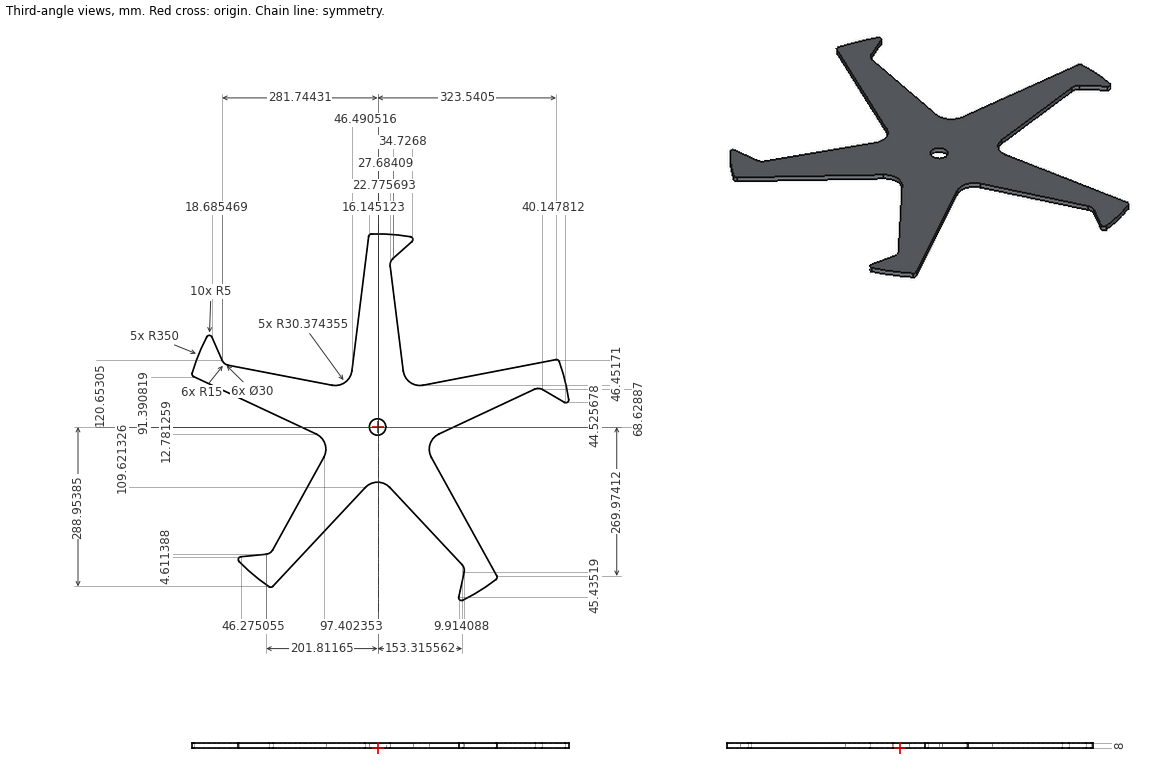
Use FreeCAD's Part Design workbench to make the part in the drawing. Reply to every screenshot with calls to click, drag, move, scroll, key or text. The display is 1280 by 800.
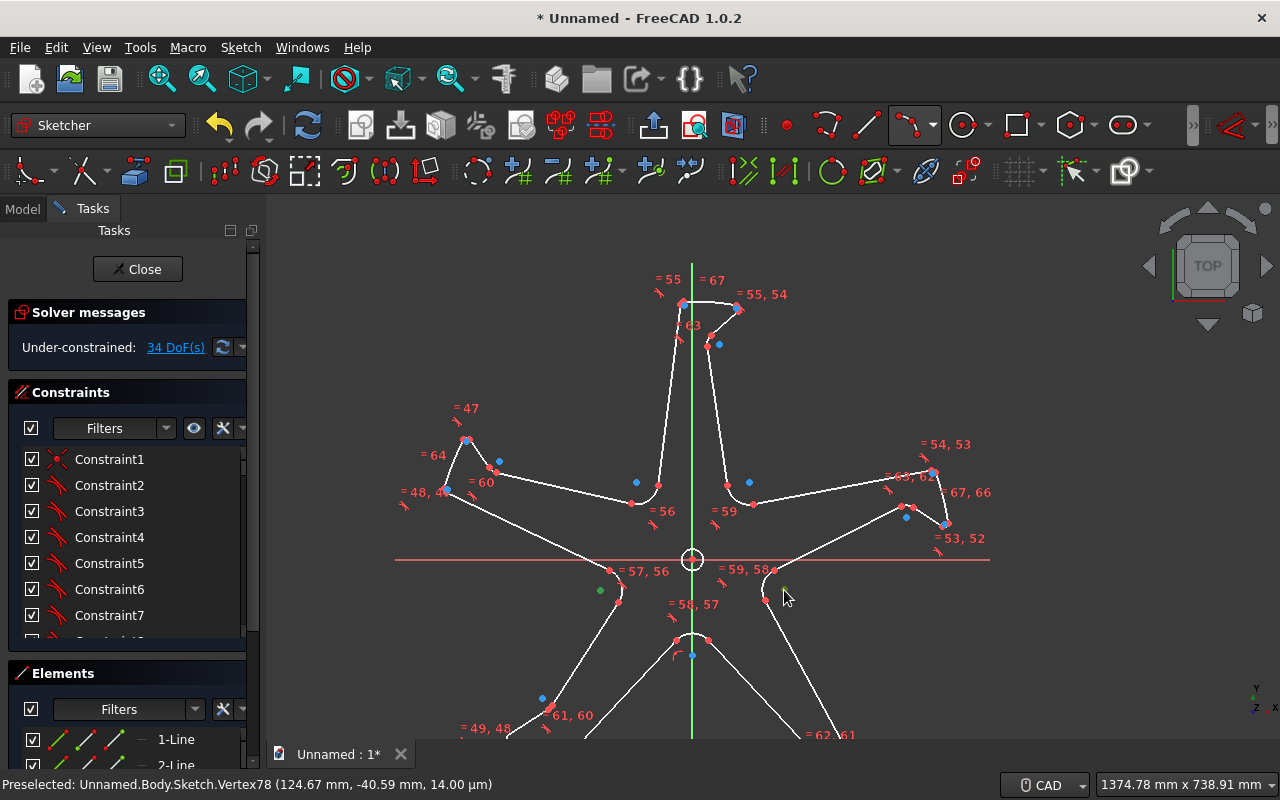
click(692, 676)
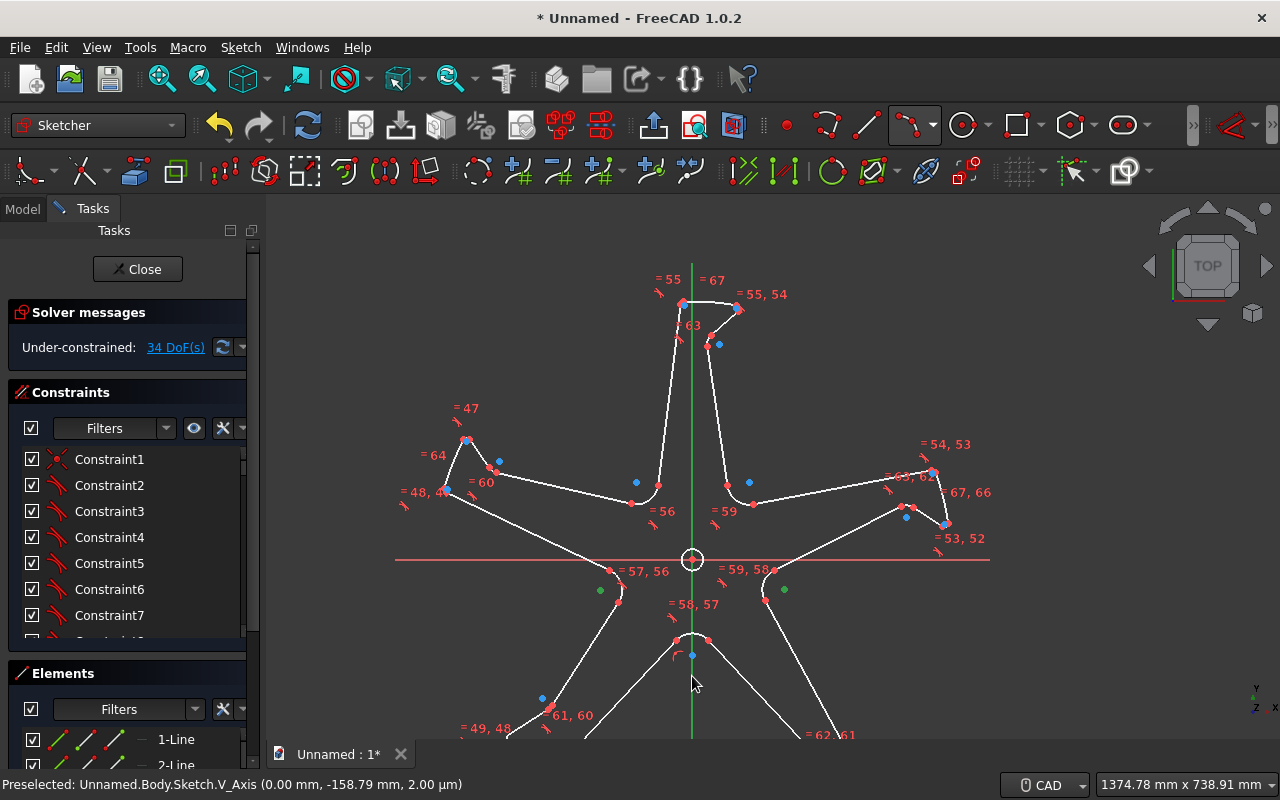
key(s)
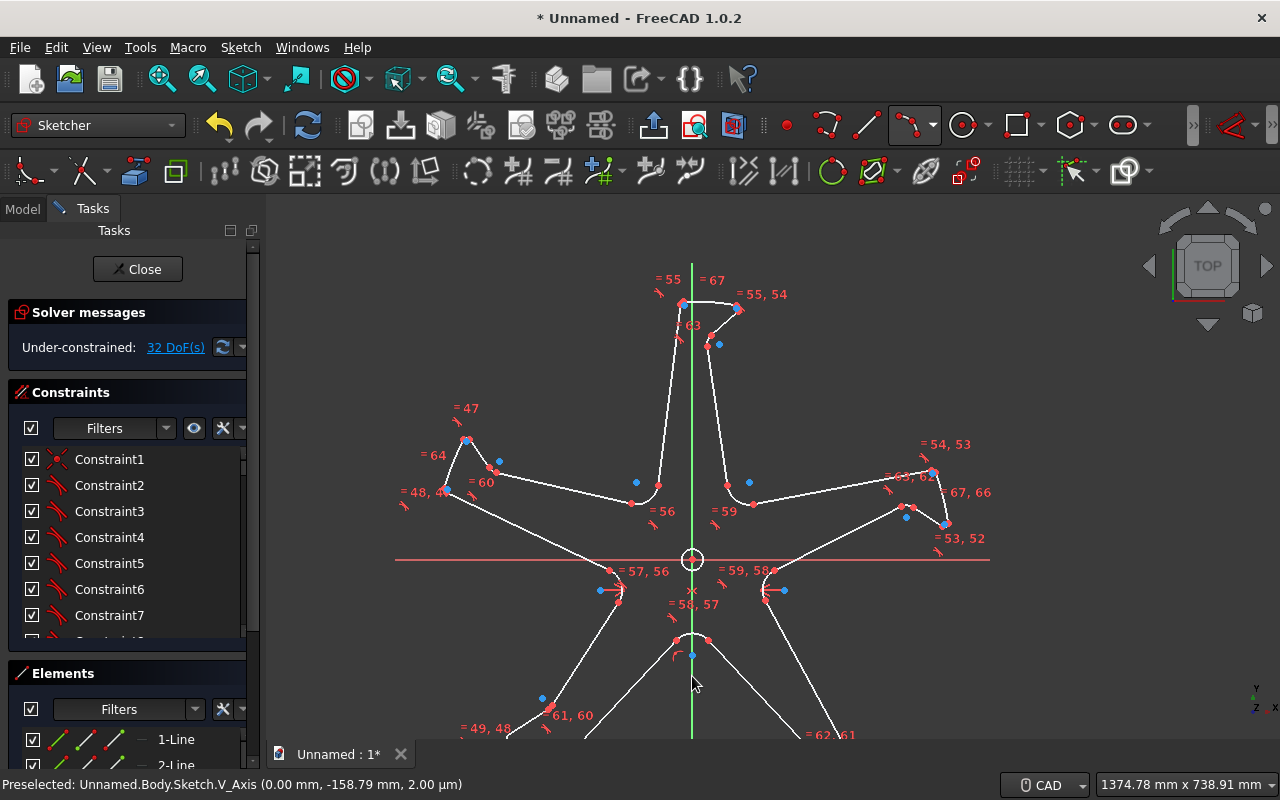
click(636, 482)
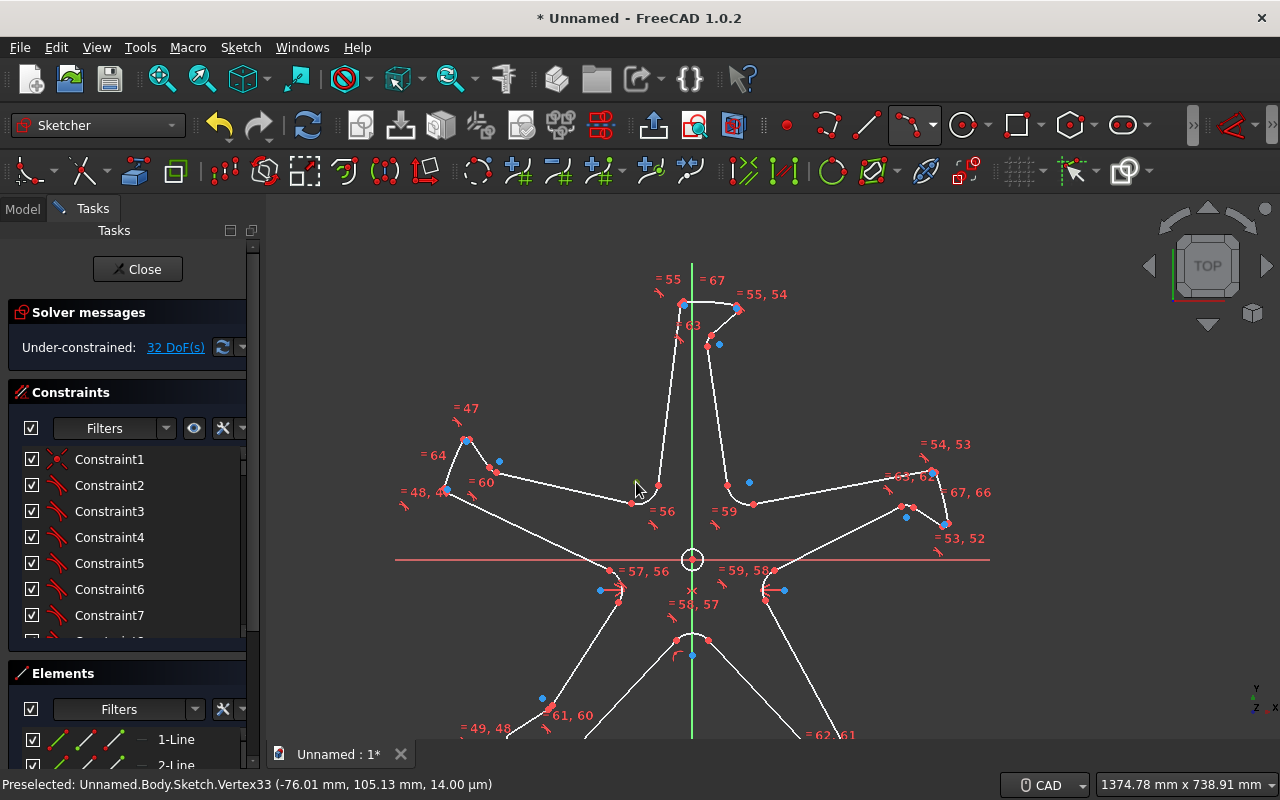
click(749, 483)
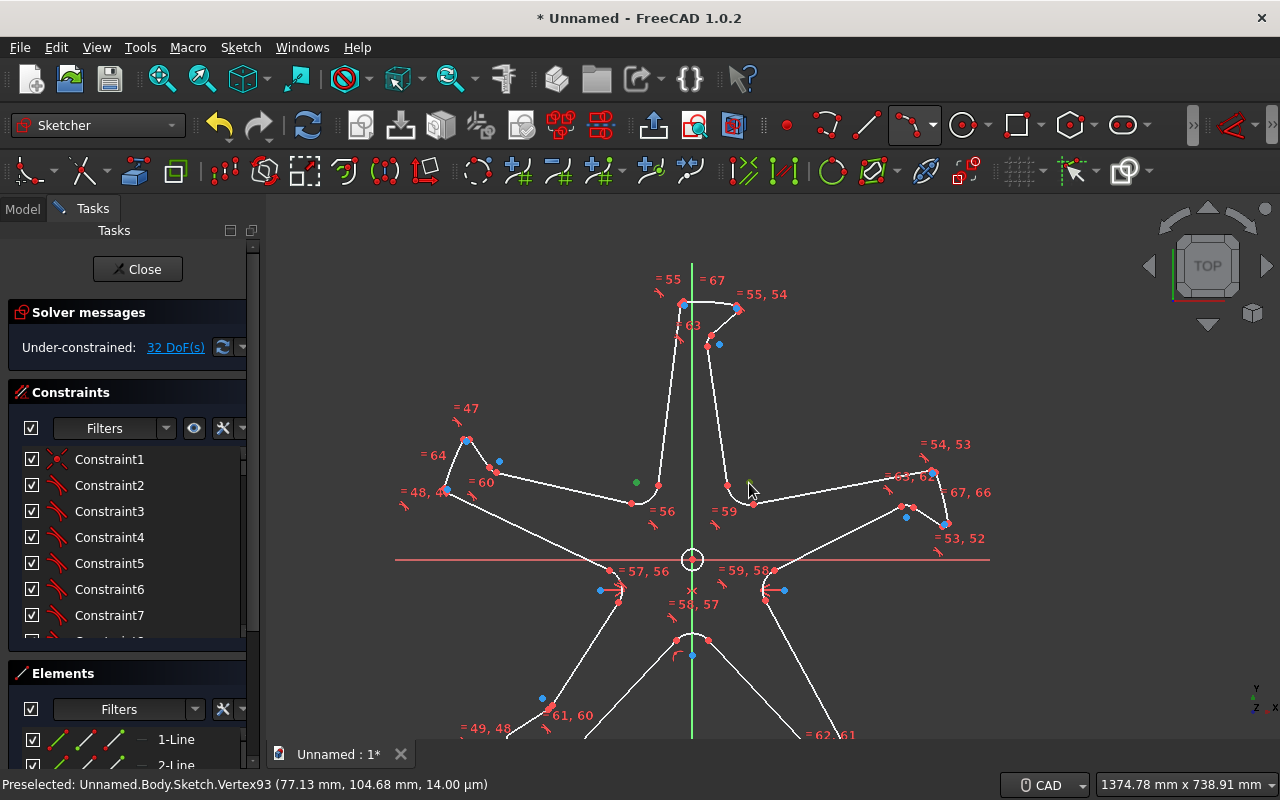
click(692, 676)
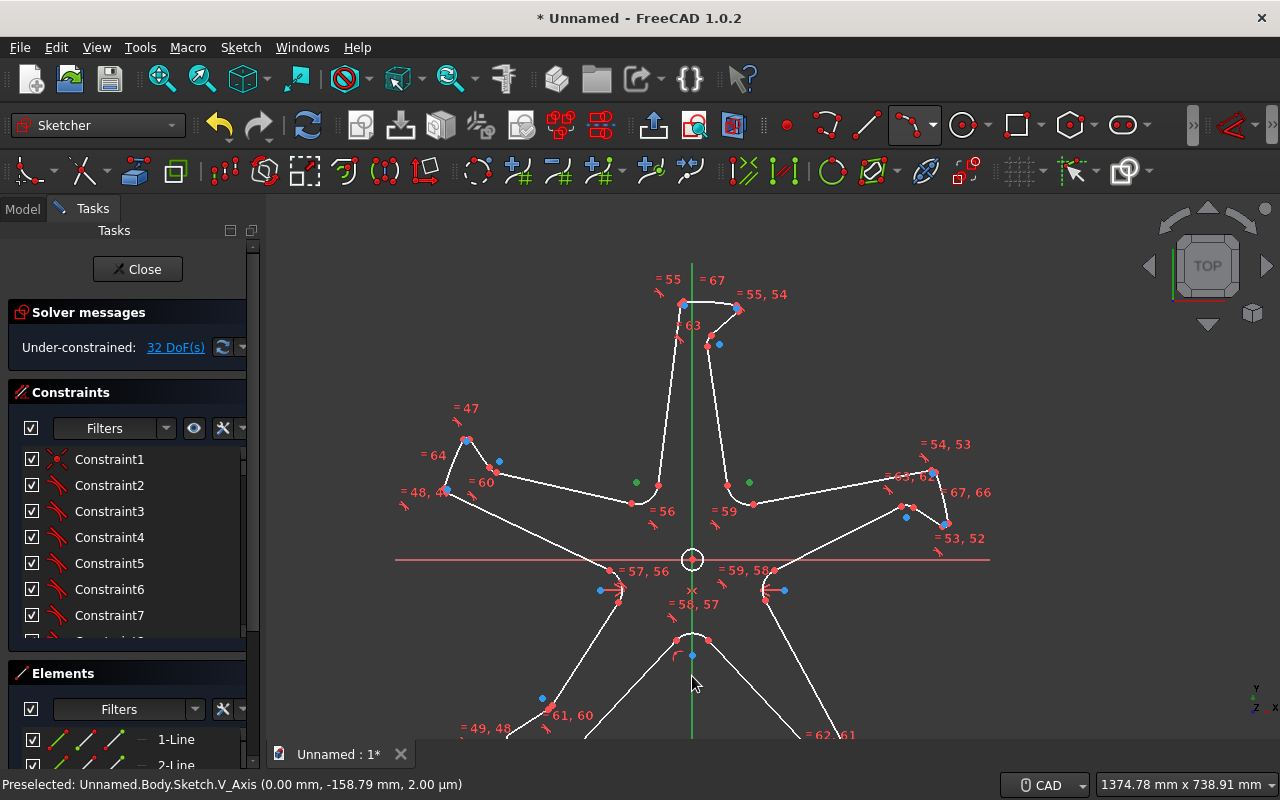
key(s)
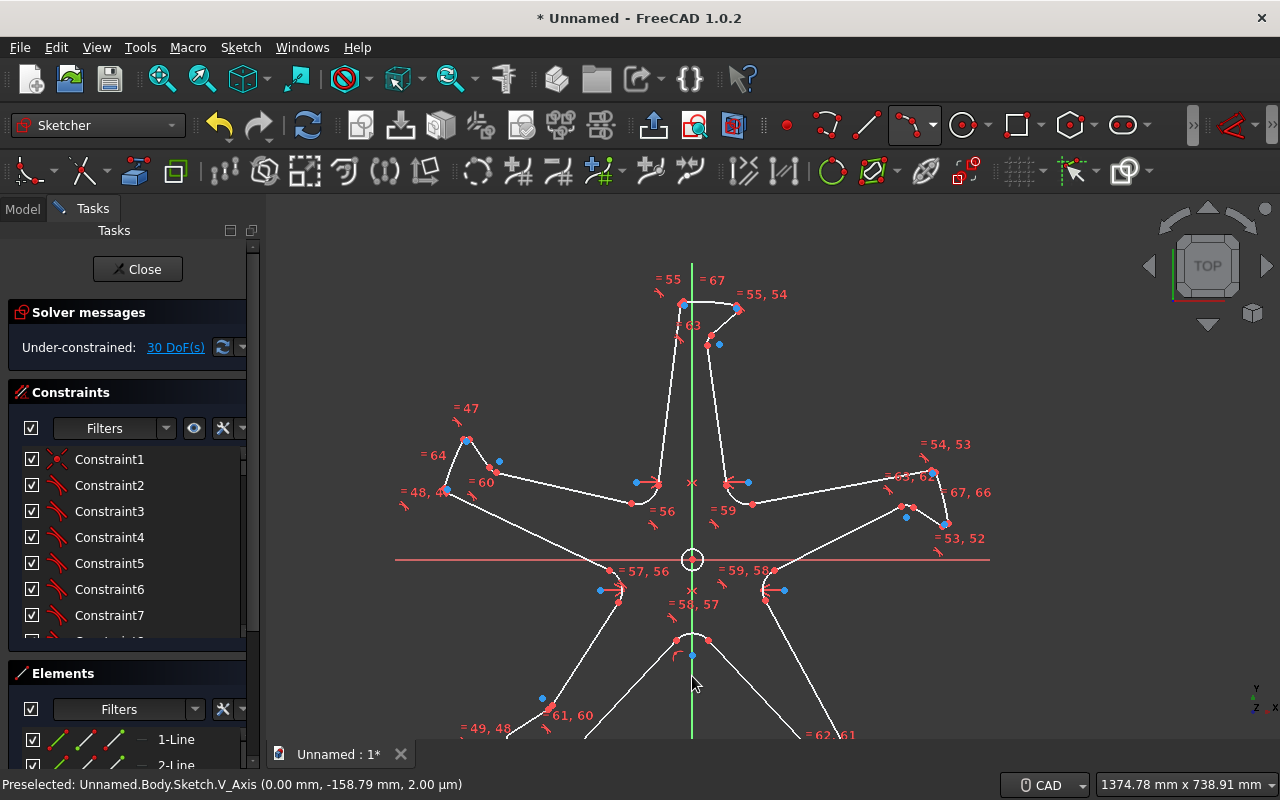
scroll(642, 504, up, 3)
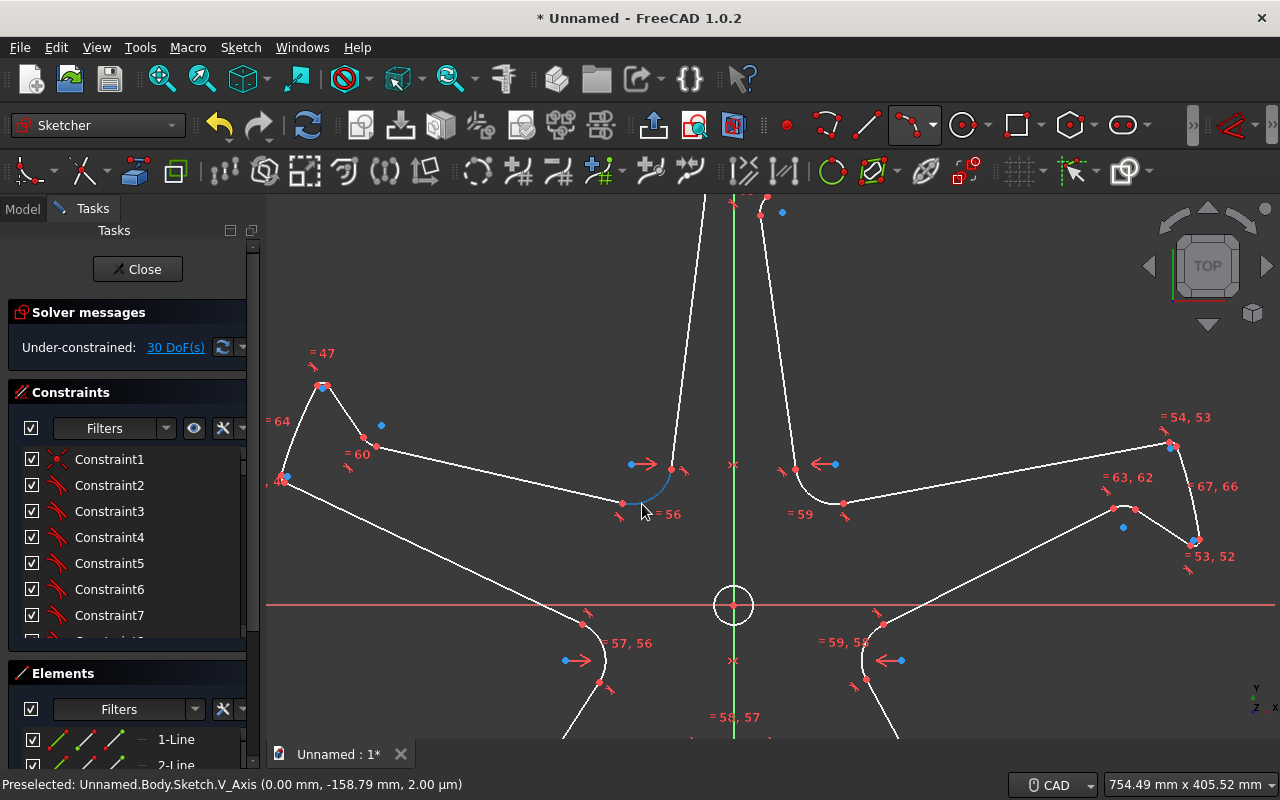
click(642, 503)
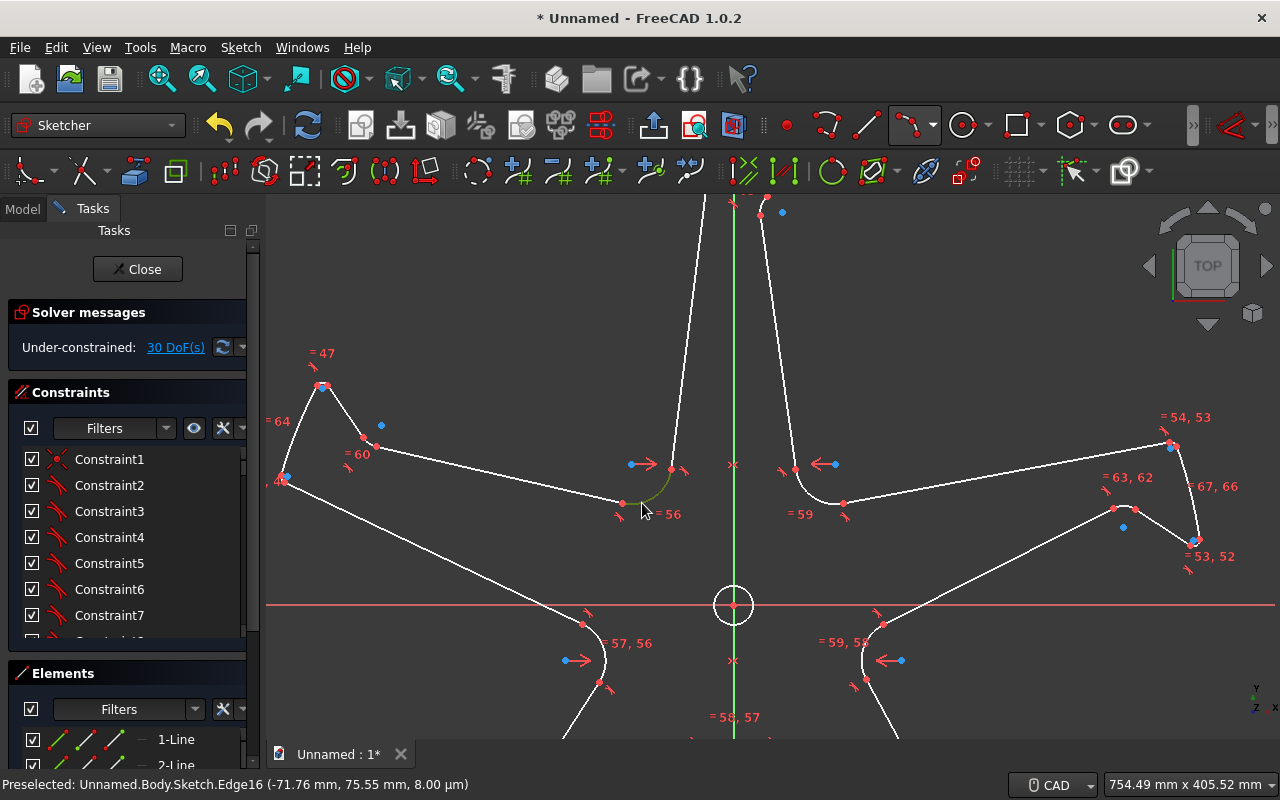
click(1258, 126)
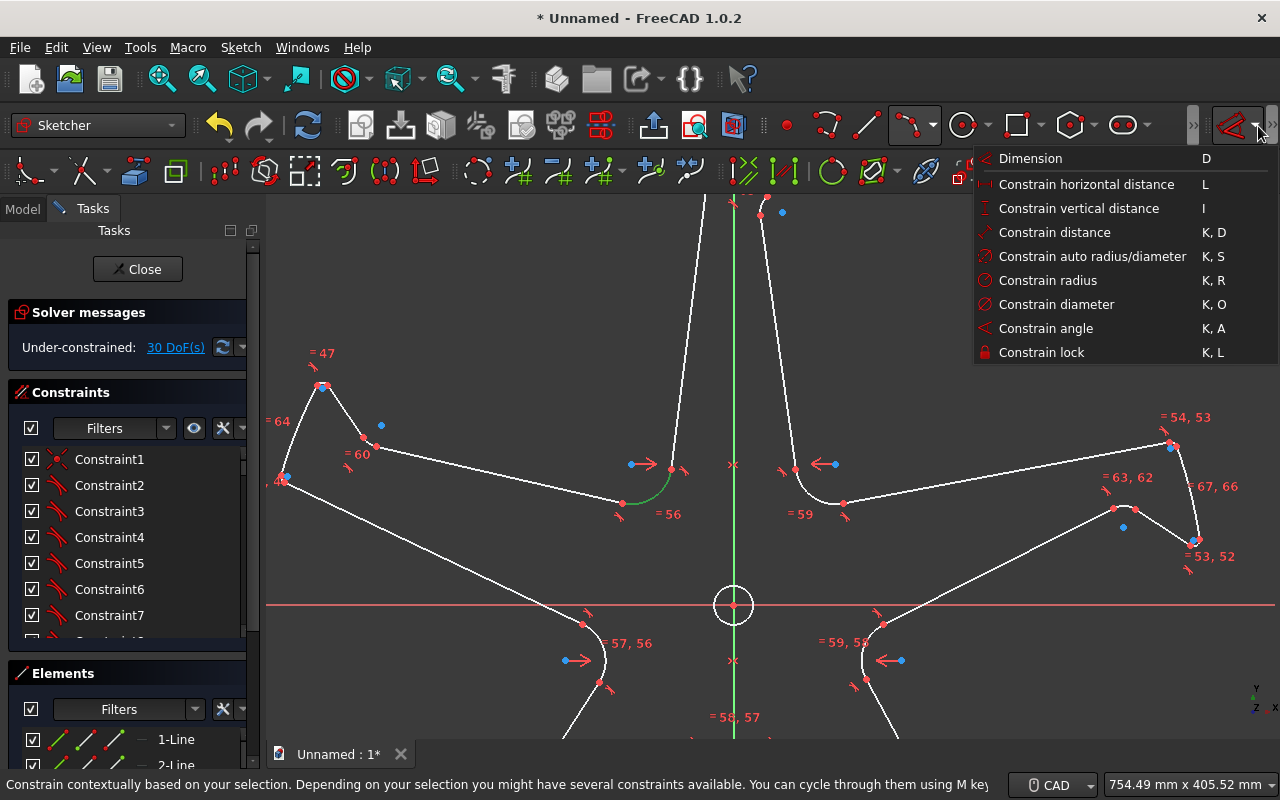
click(1126, 280)